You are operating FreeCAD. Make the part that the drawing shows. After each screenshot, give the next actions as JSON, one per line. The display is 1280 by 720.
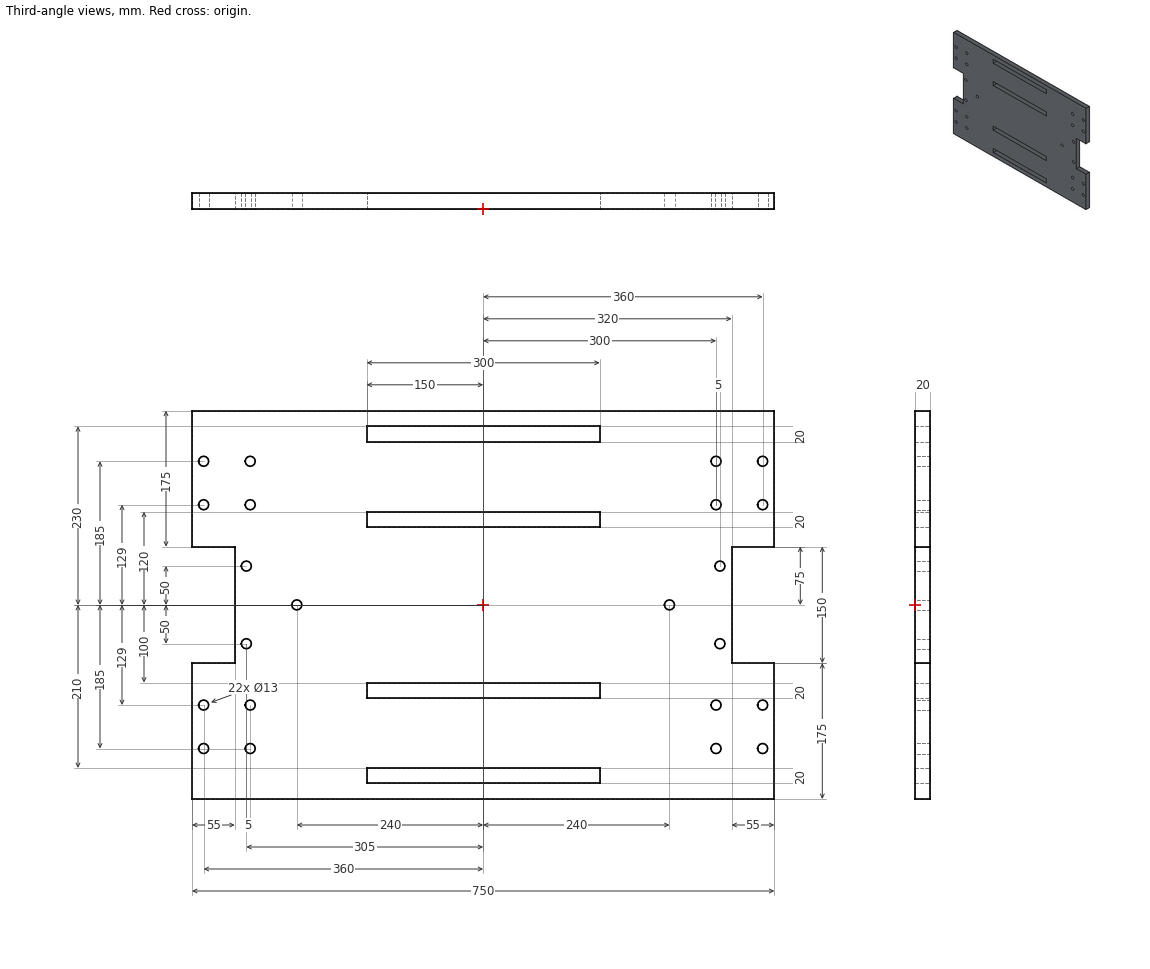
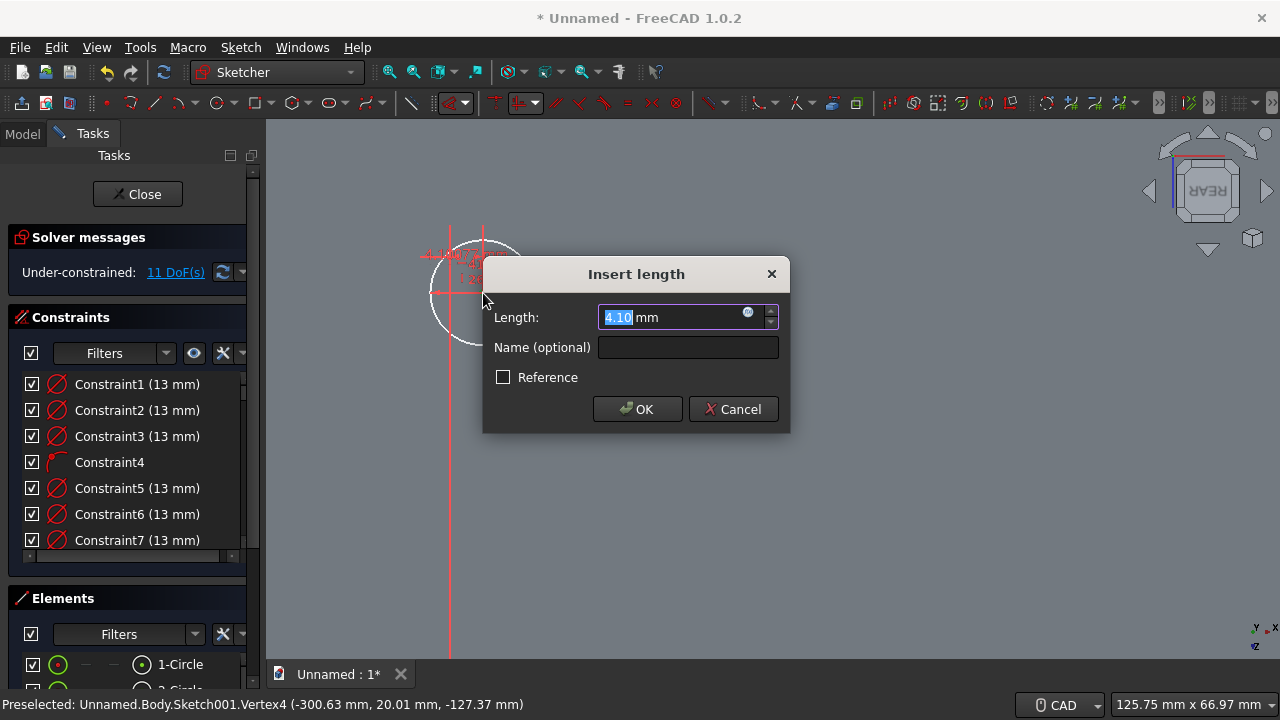
{"action": "type", "text": "5"}
{"action": "key", "text": "Return"}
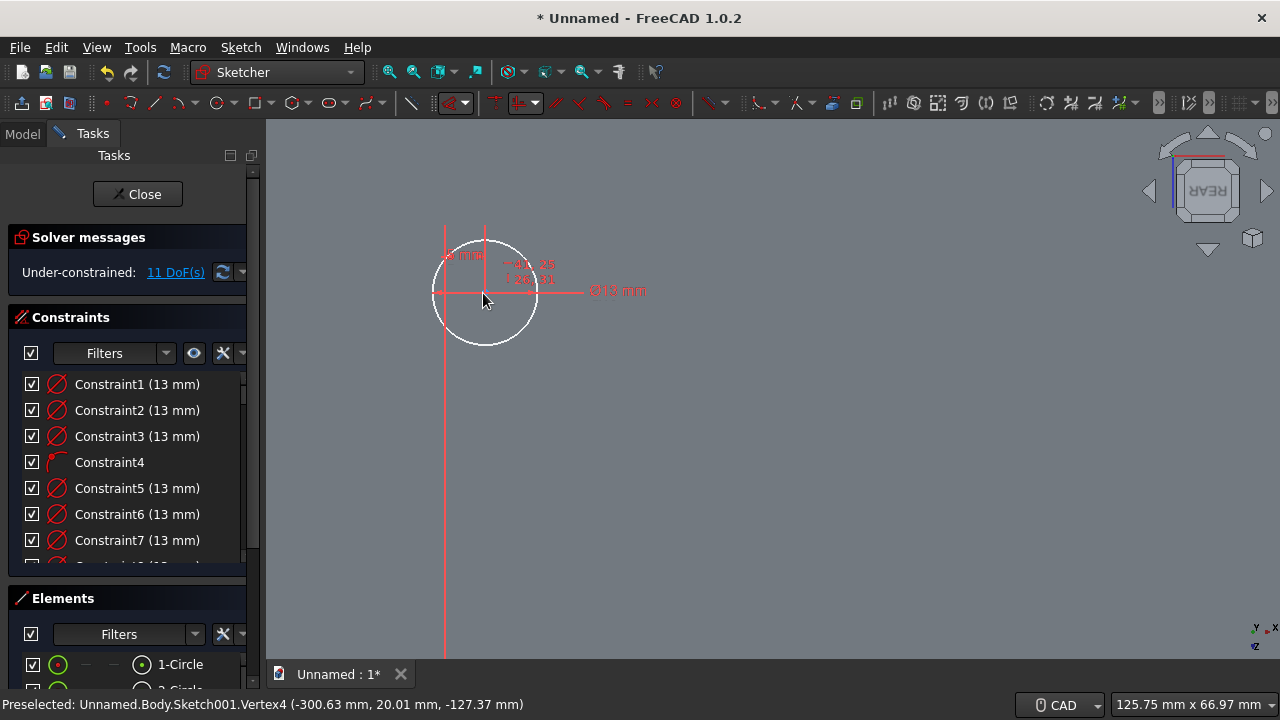
{"action": "scroll", "coordinate": [485, 296], "scroll_direction": "down", "scroll_amount": 12}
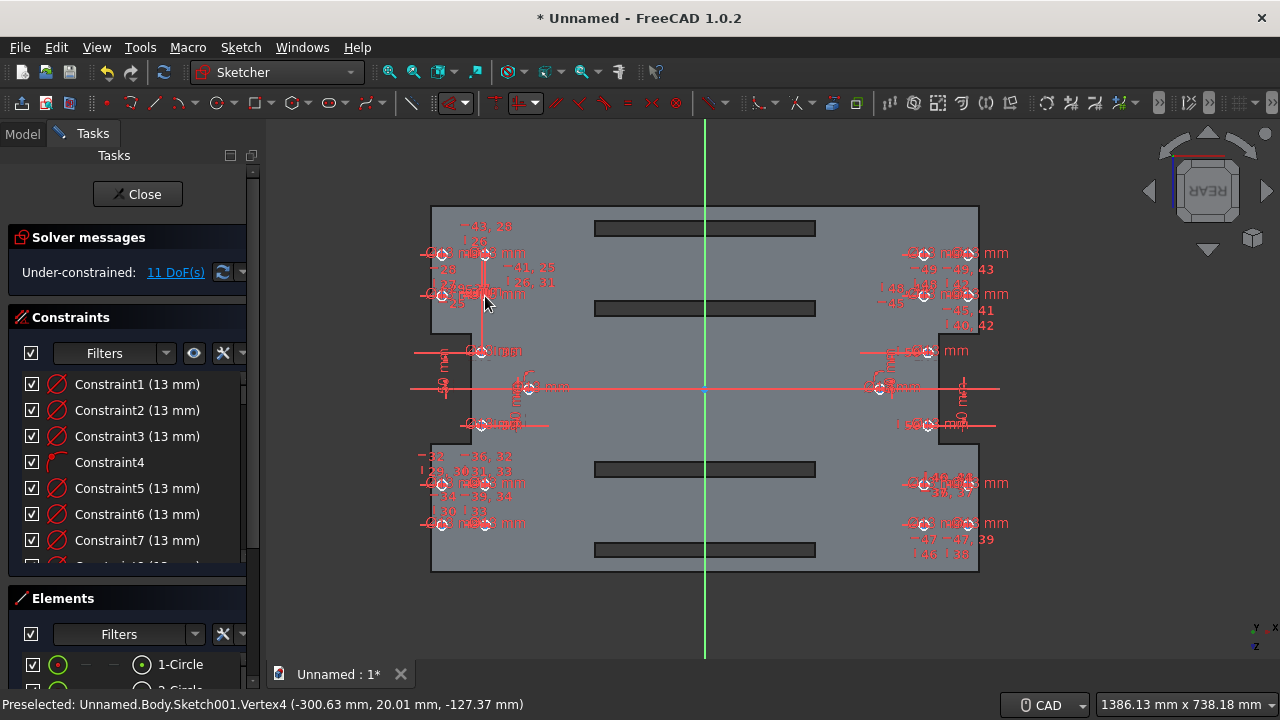
{"action": "scroll", "coordinate": [924, 485], "scroll_direction": "up", "scroll_amount": 12}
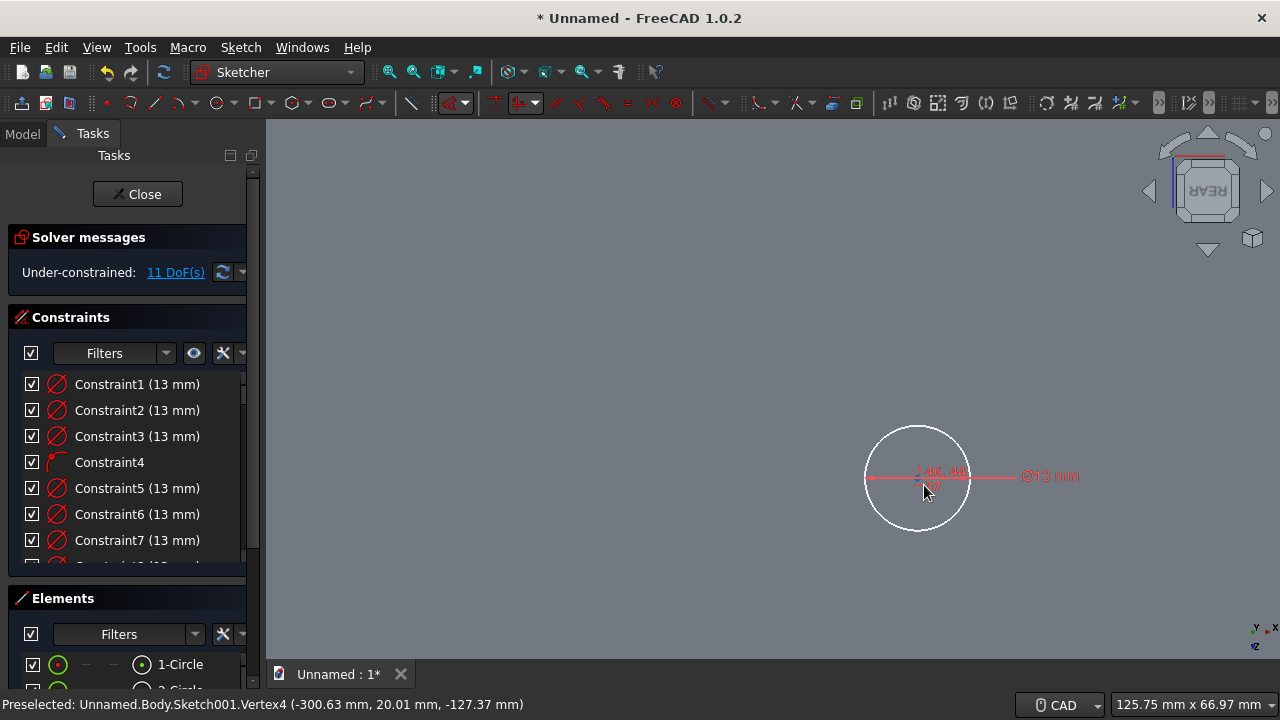
{"action": "left_click", "coordinate": [917, 478]}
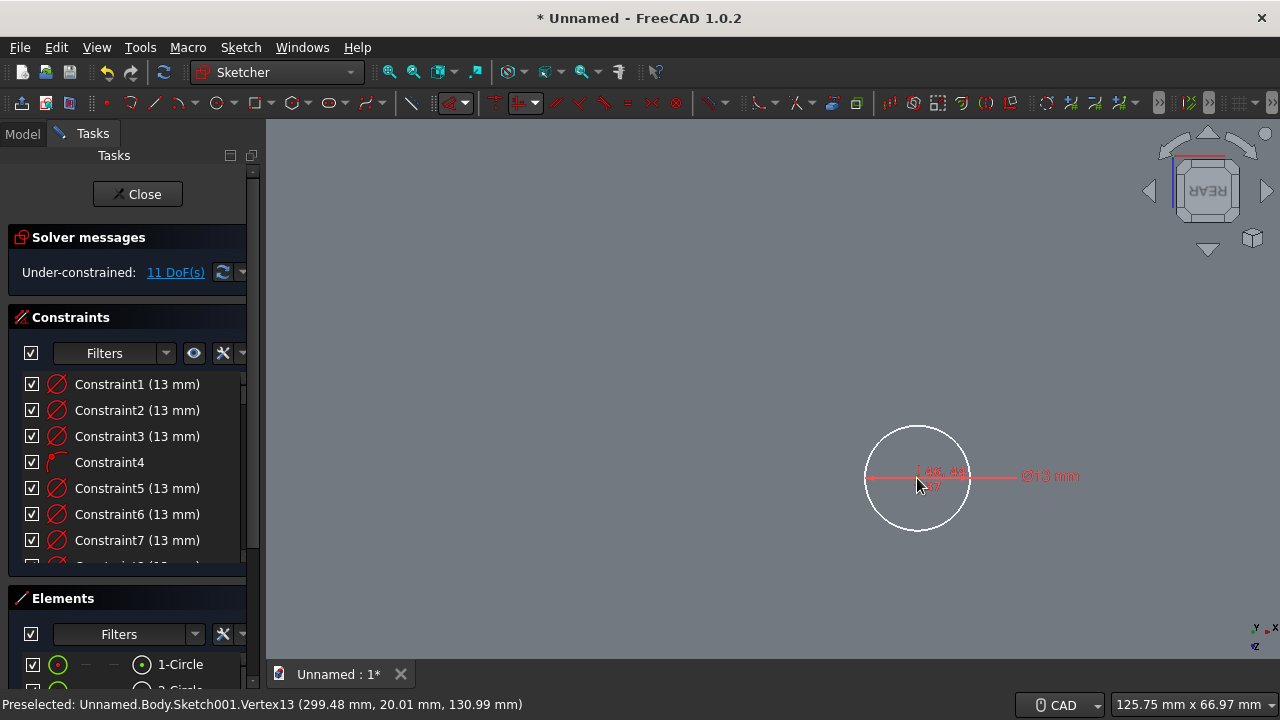
{"action": "scroll", "coordinate": [924, 485], "scroll_direction": "down", "scroll_amount": 12}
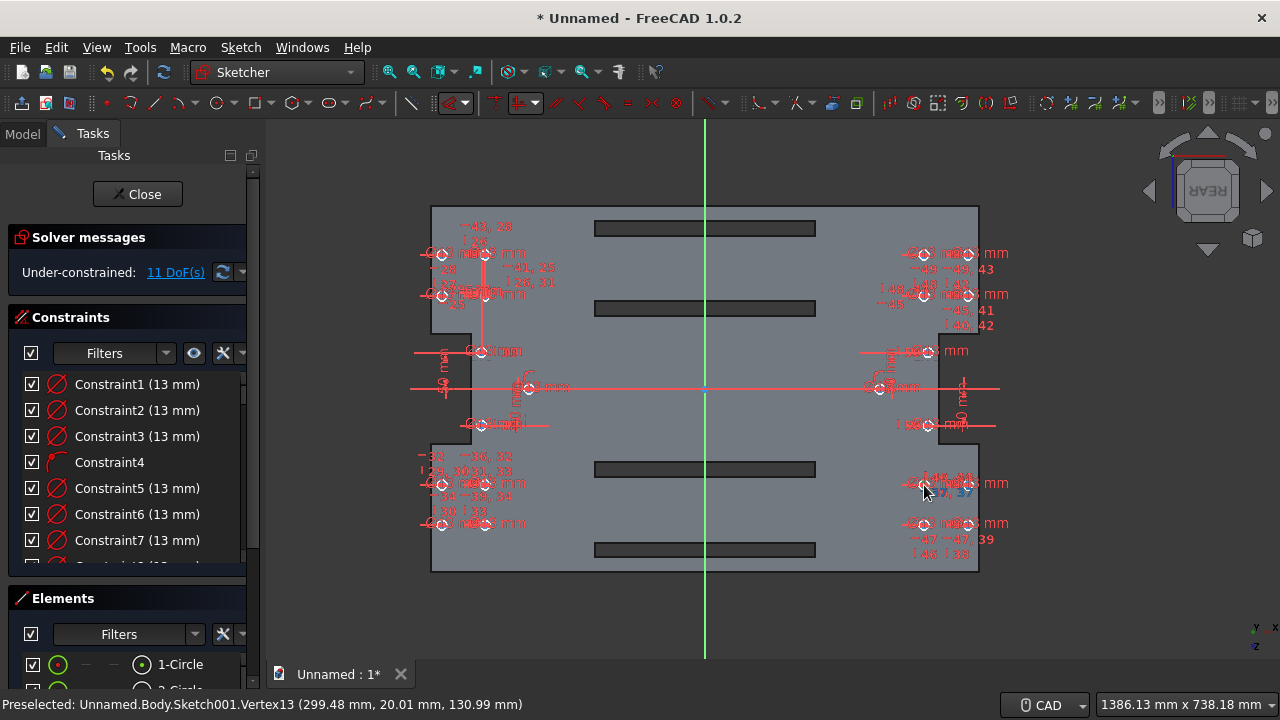
{"action": "scroll", "coordinate": [928, 426], "scroll_direction": "up", "scroll_amount": 12}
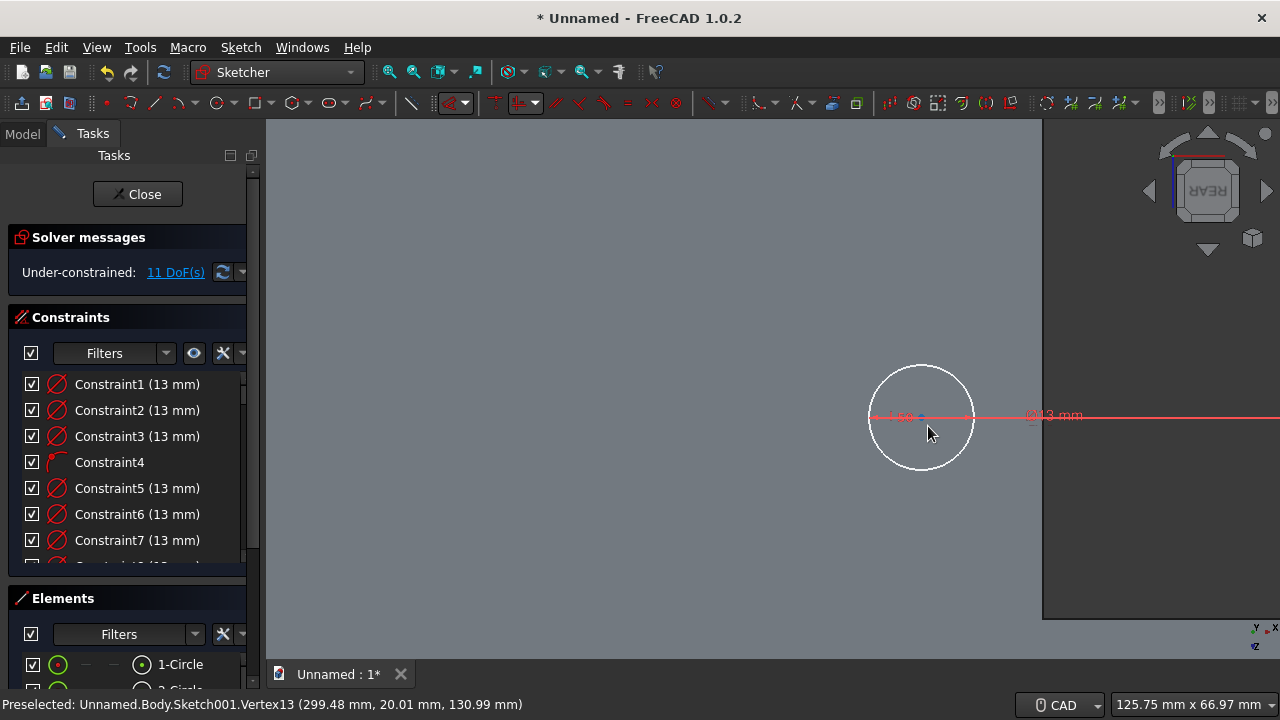
{"action": "left_click", "coordinate": [921, 418]}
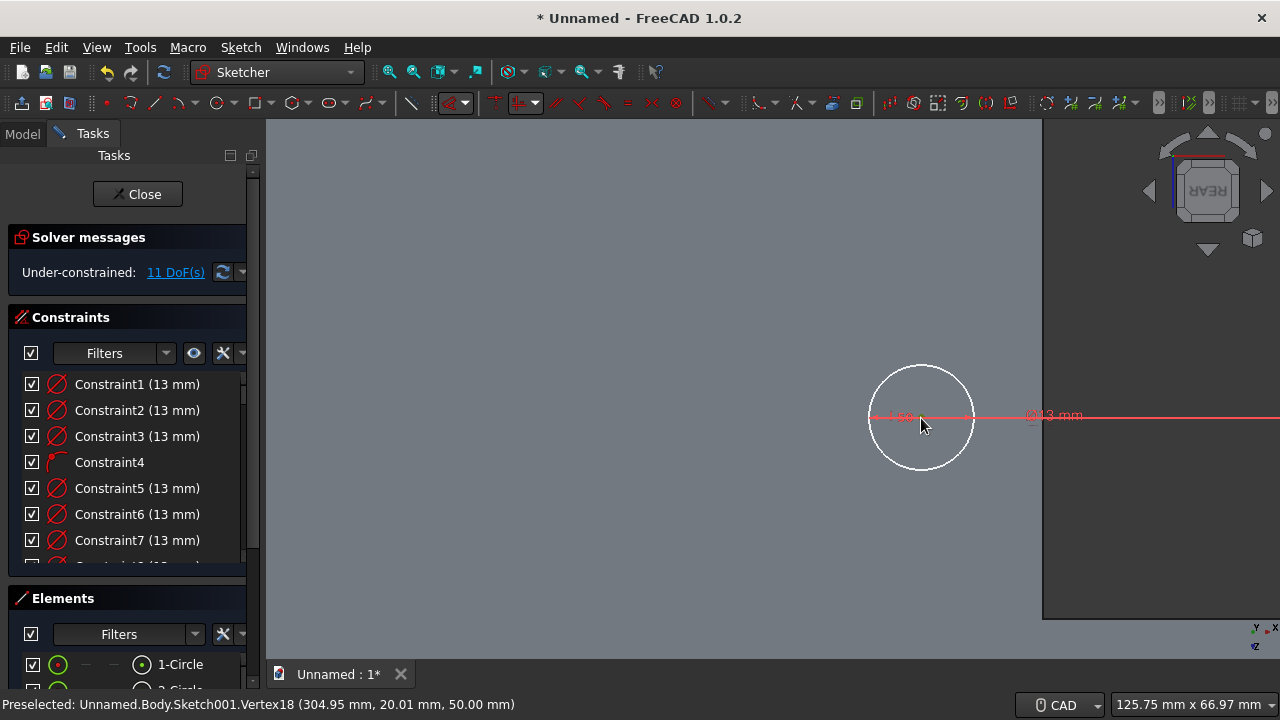
{"action": "key", "text": "l"}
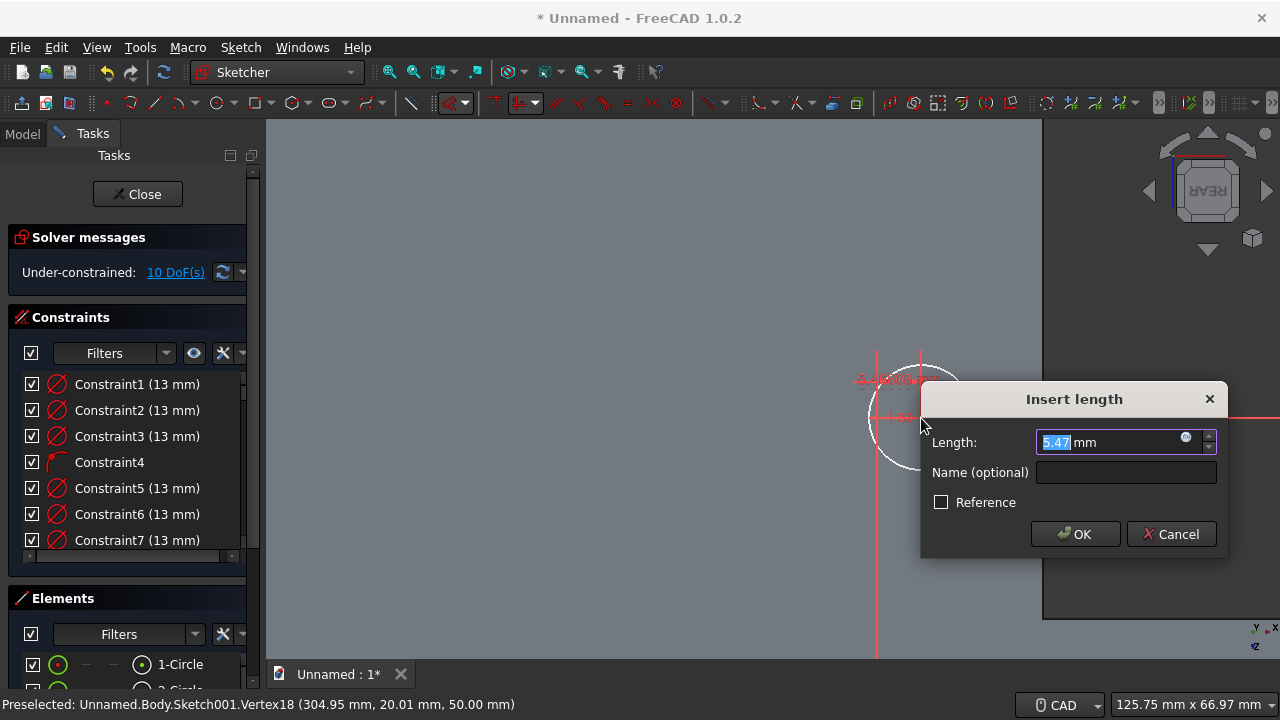
{"action": "type", "text": "5"}
{"action": "key", "text": "Return"}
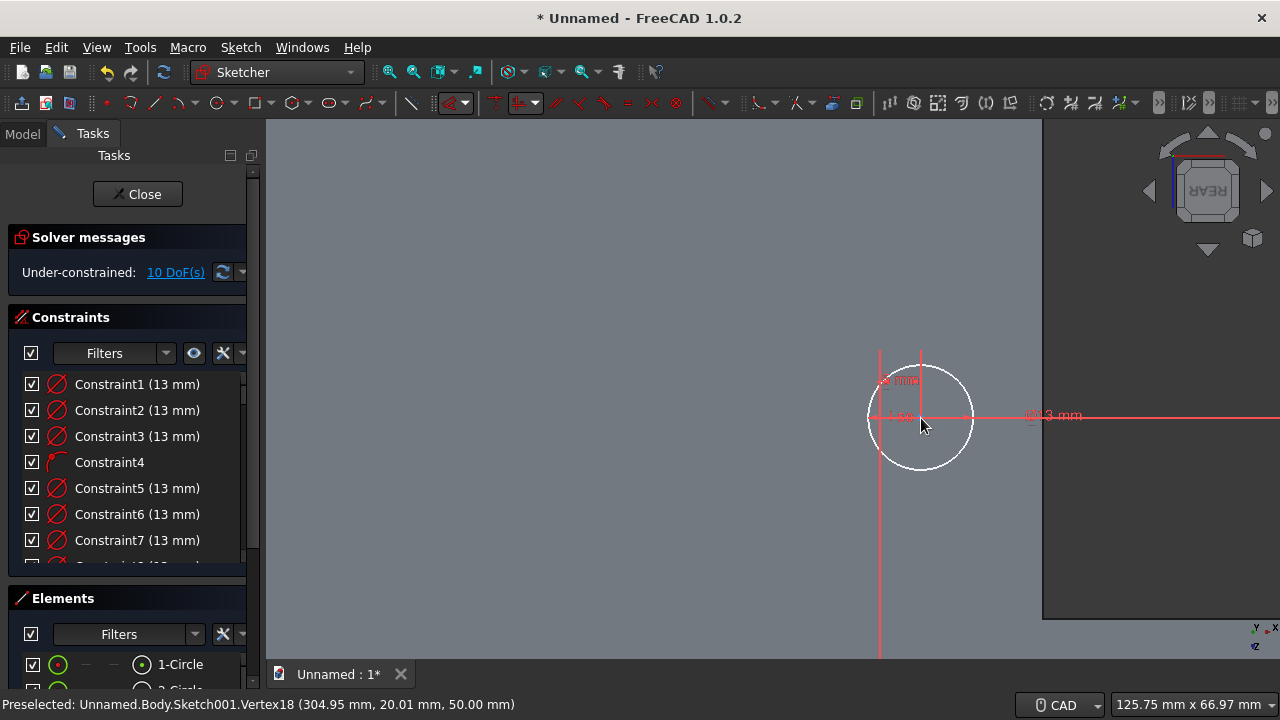
{"action": "scroll", "coordinate": [928, 426], "scroll_direction": "down", "scroll_amount": 12}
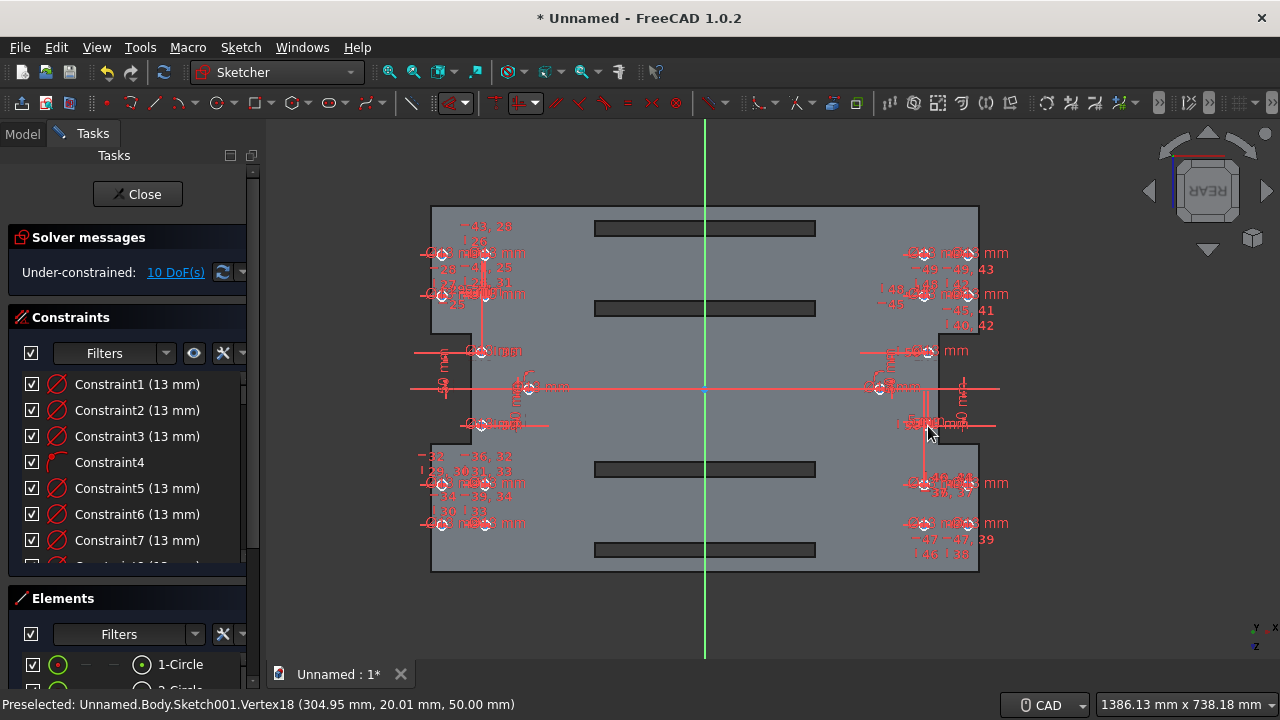
{"action": "left_click", "coordinate": [442, 296]}